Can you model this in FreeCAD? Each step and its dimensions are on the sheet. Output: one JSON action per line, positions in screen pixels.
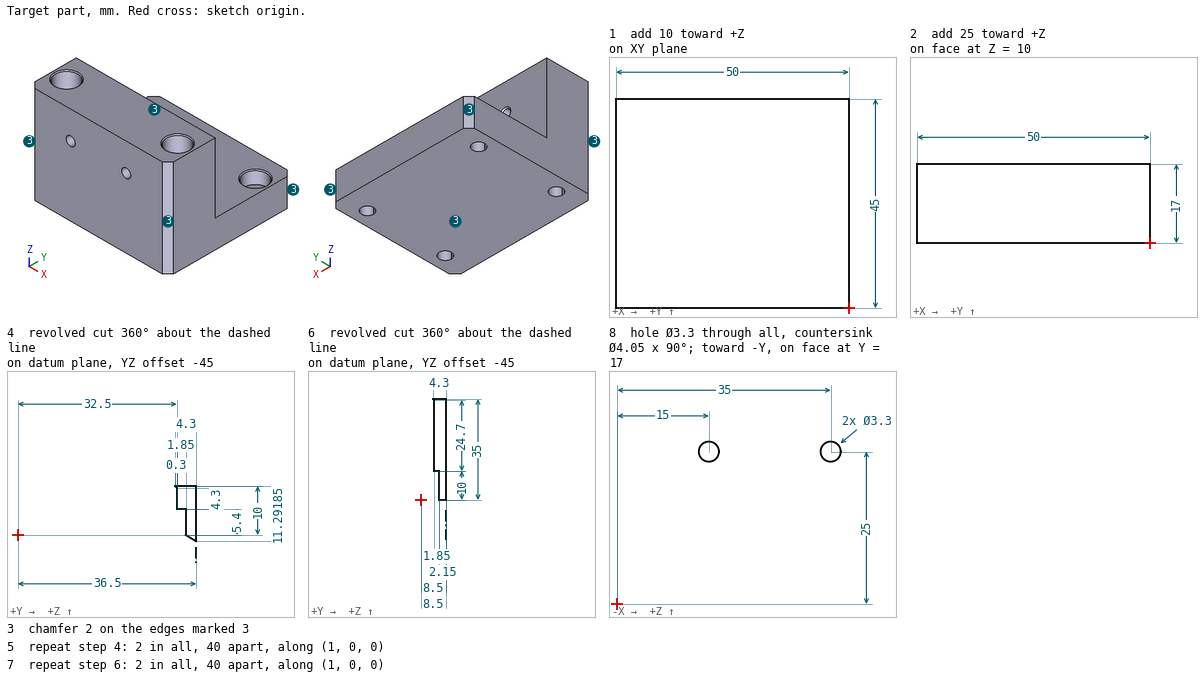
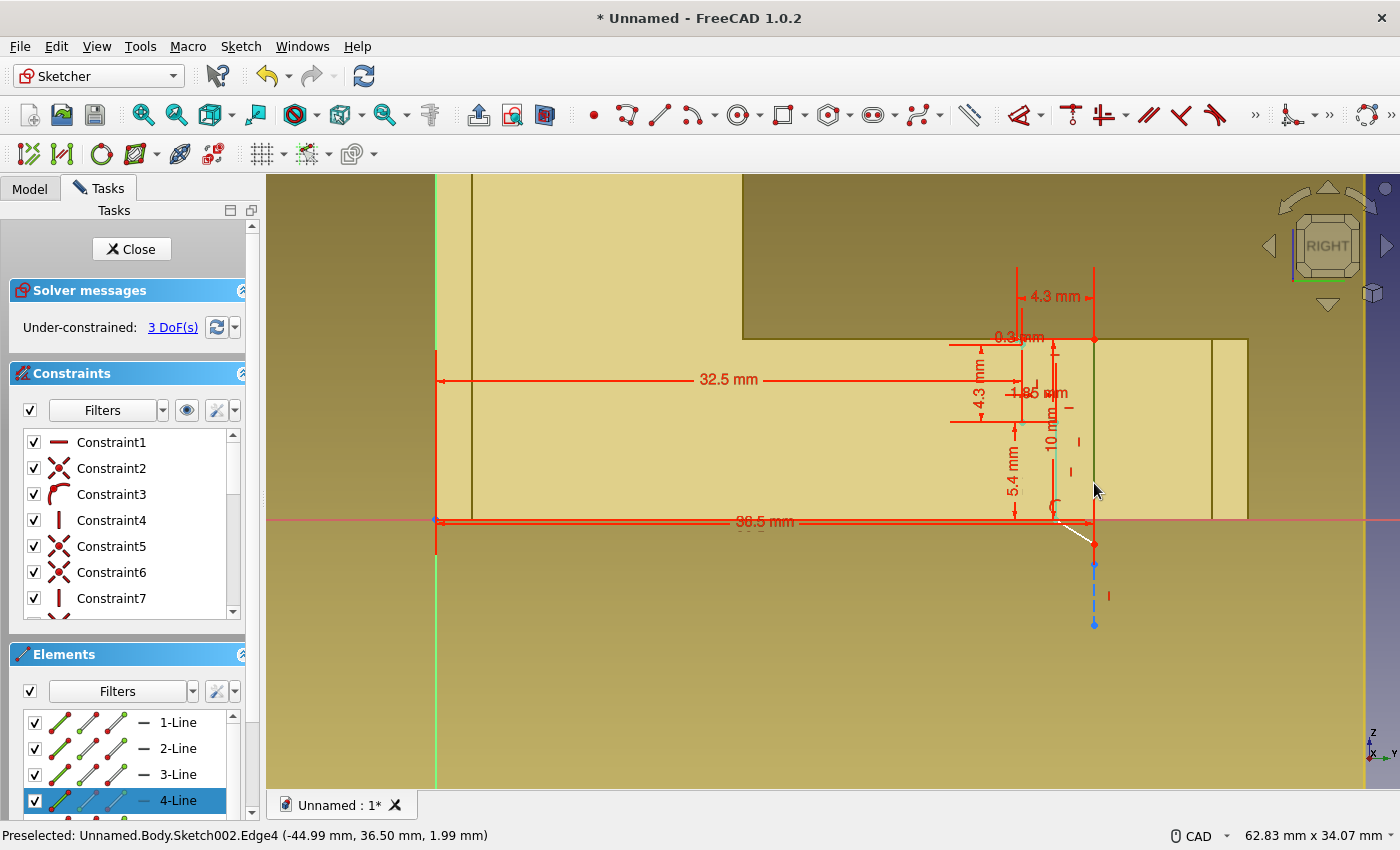
{"action": "left_click", "coordinate": [1040, 116]}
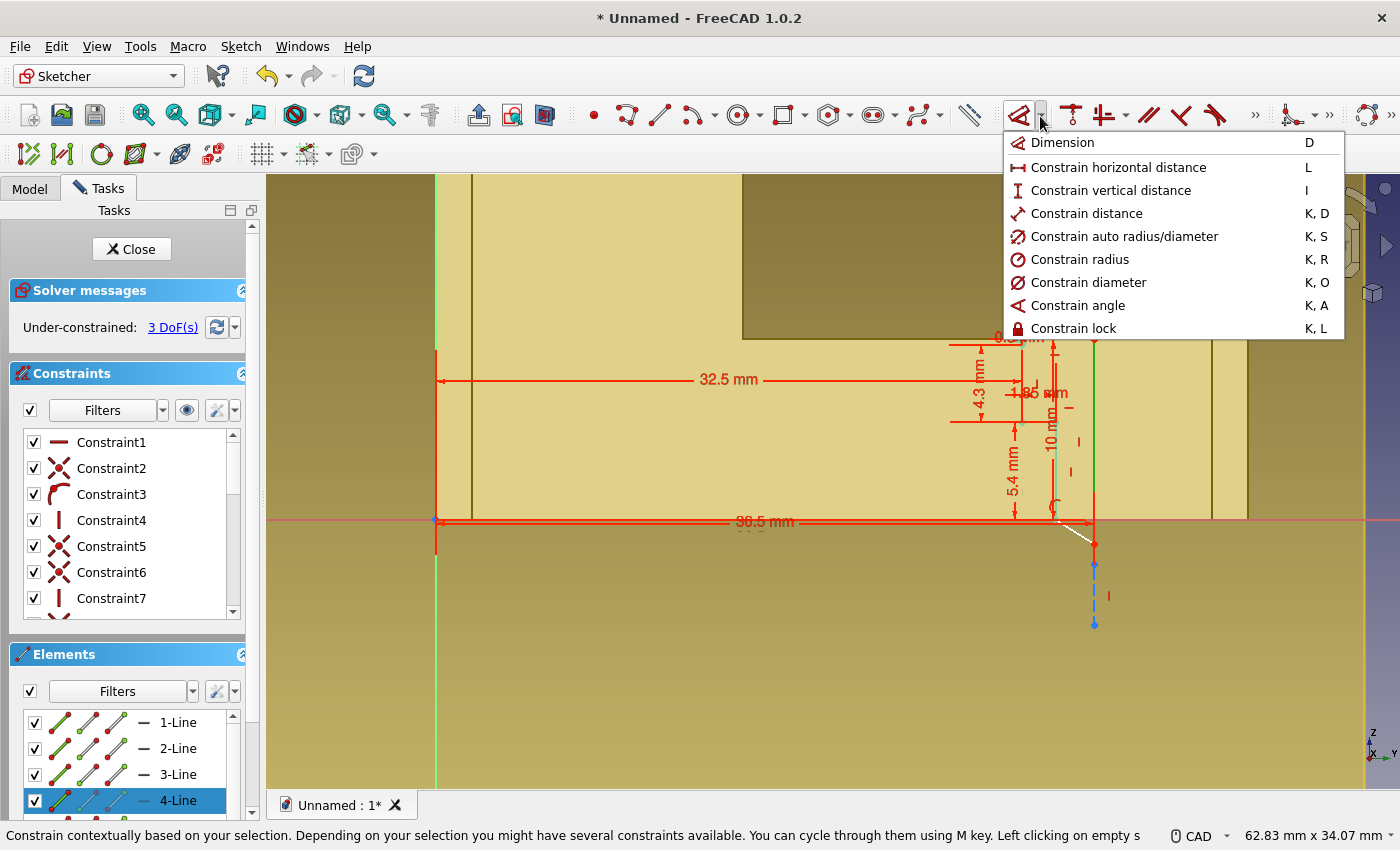
{"action": "left_click", "coordinate": [1174, 190]}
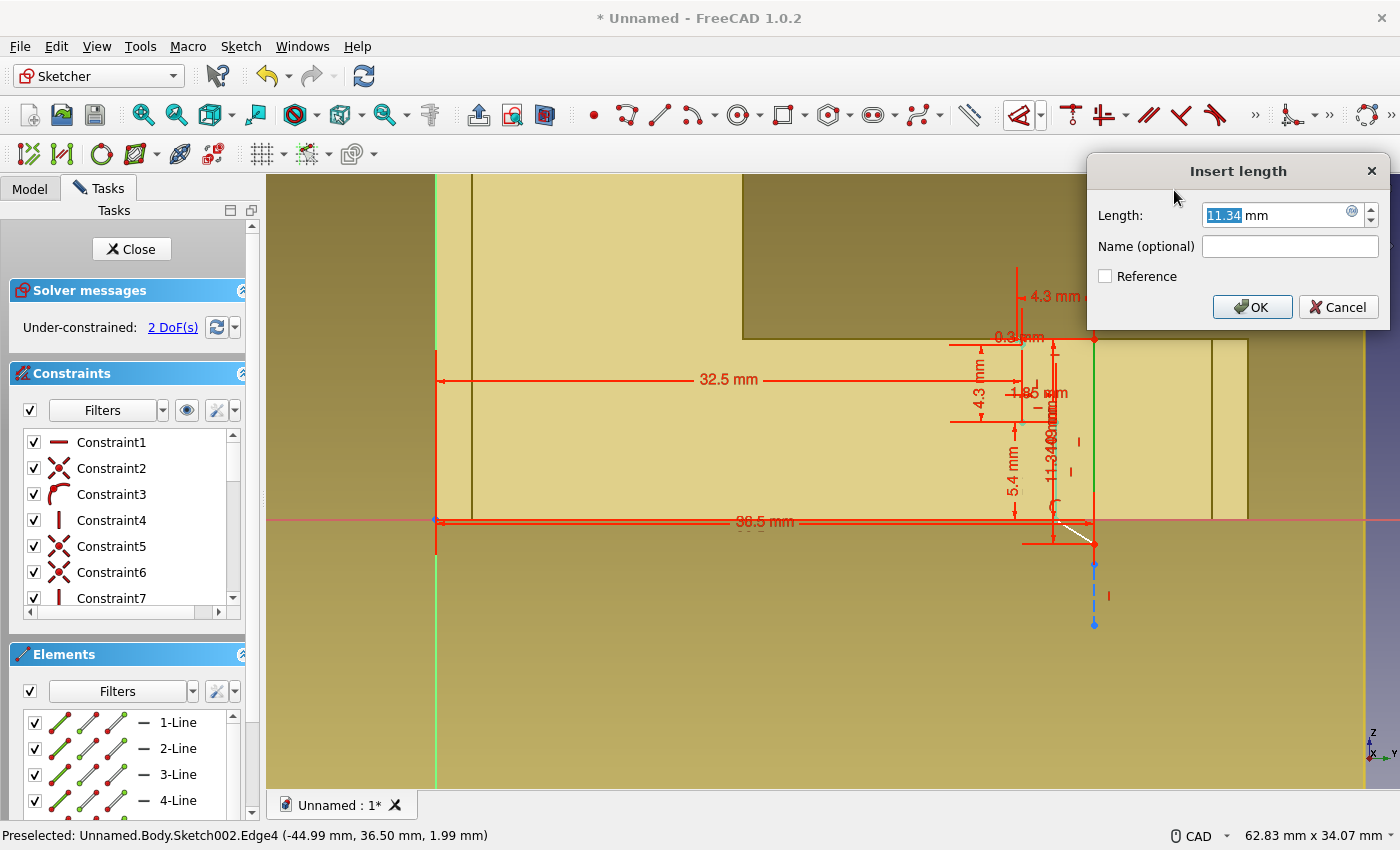
{"action": "type", "text": "11.29185"}
{"action": "key", "text": "Return"}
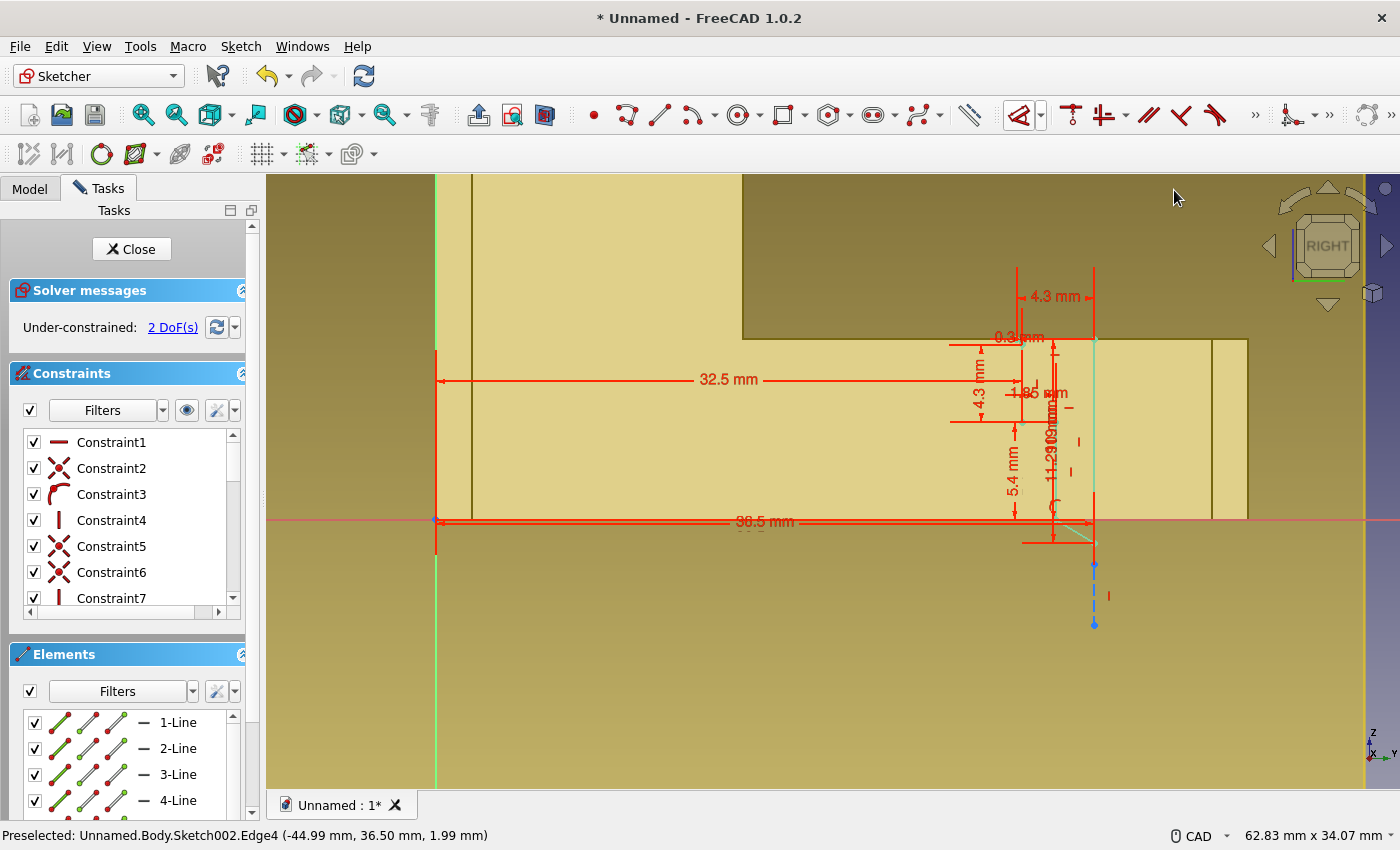
{"action": "left_click", "coordinate": [132, 249]}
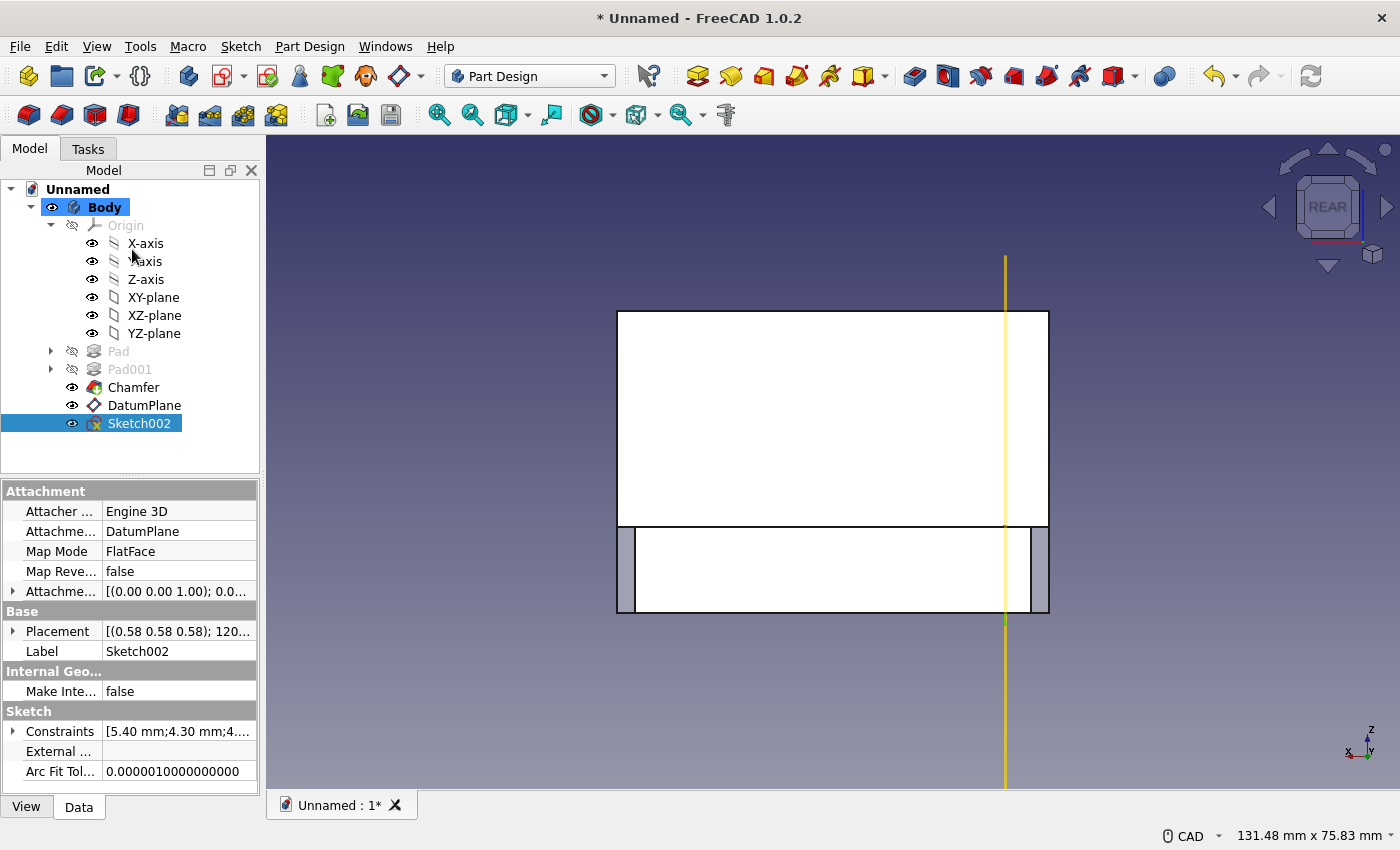
{"action": "left_click", "coordinate": [981, 76]}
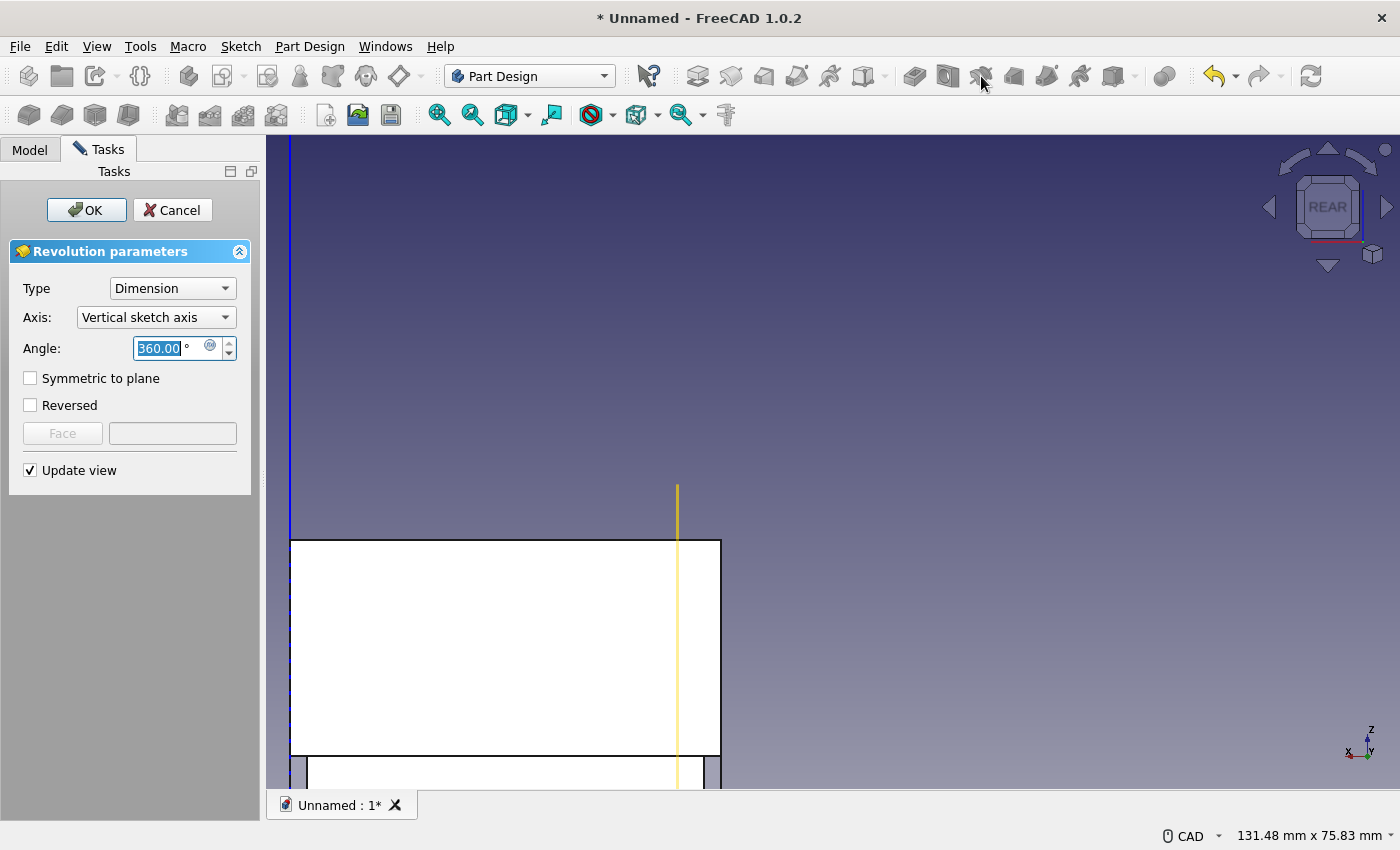
{"action": "left_click", "coordinate": [157, 318]}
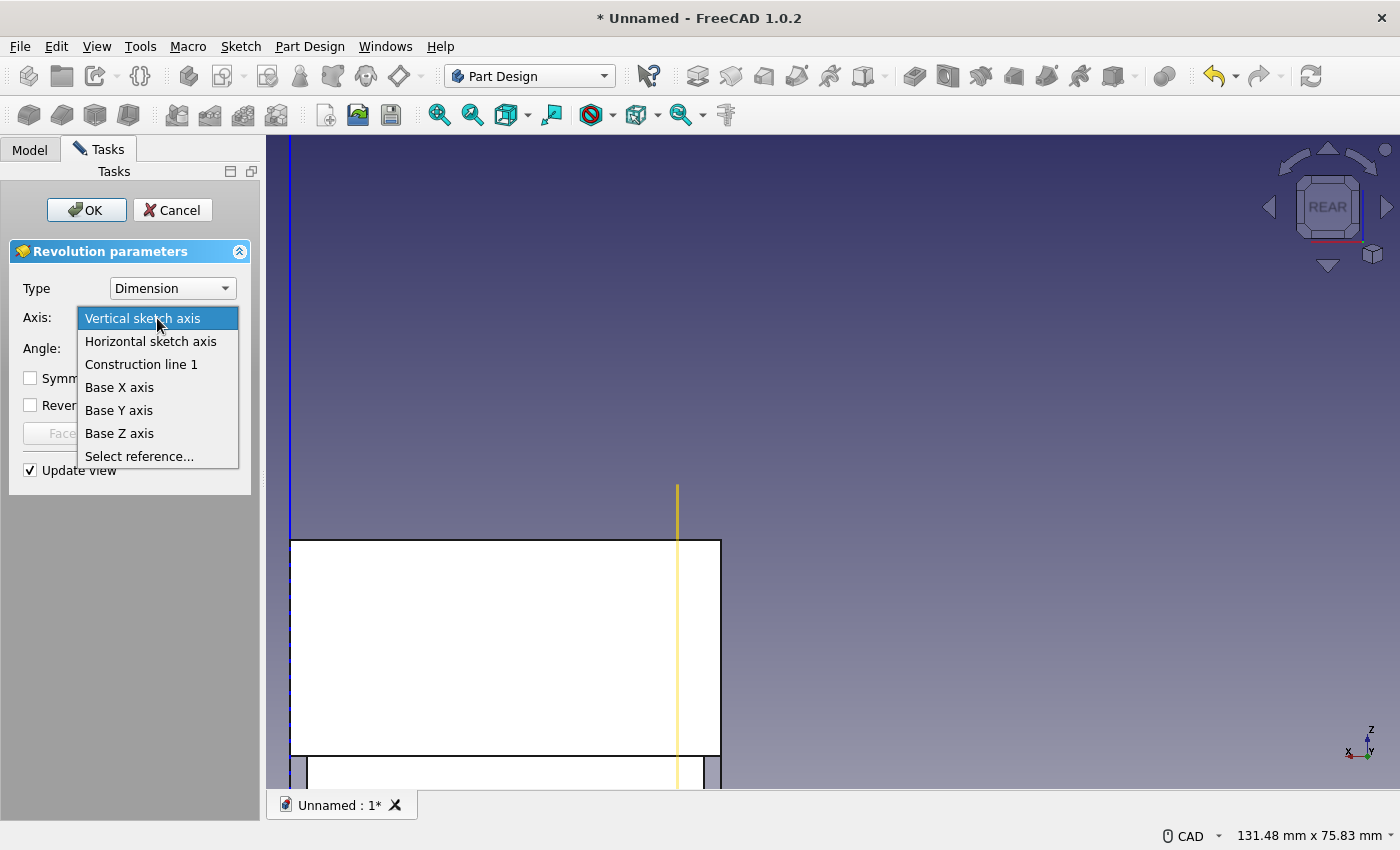
{"action": "left_click", "coordinate": [156, 364]}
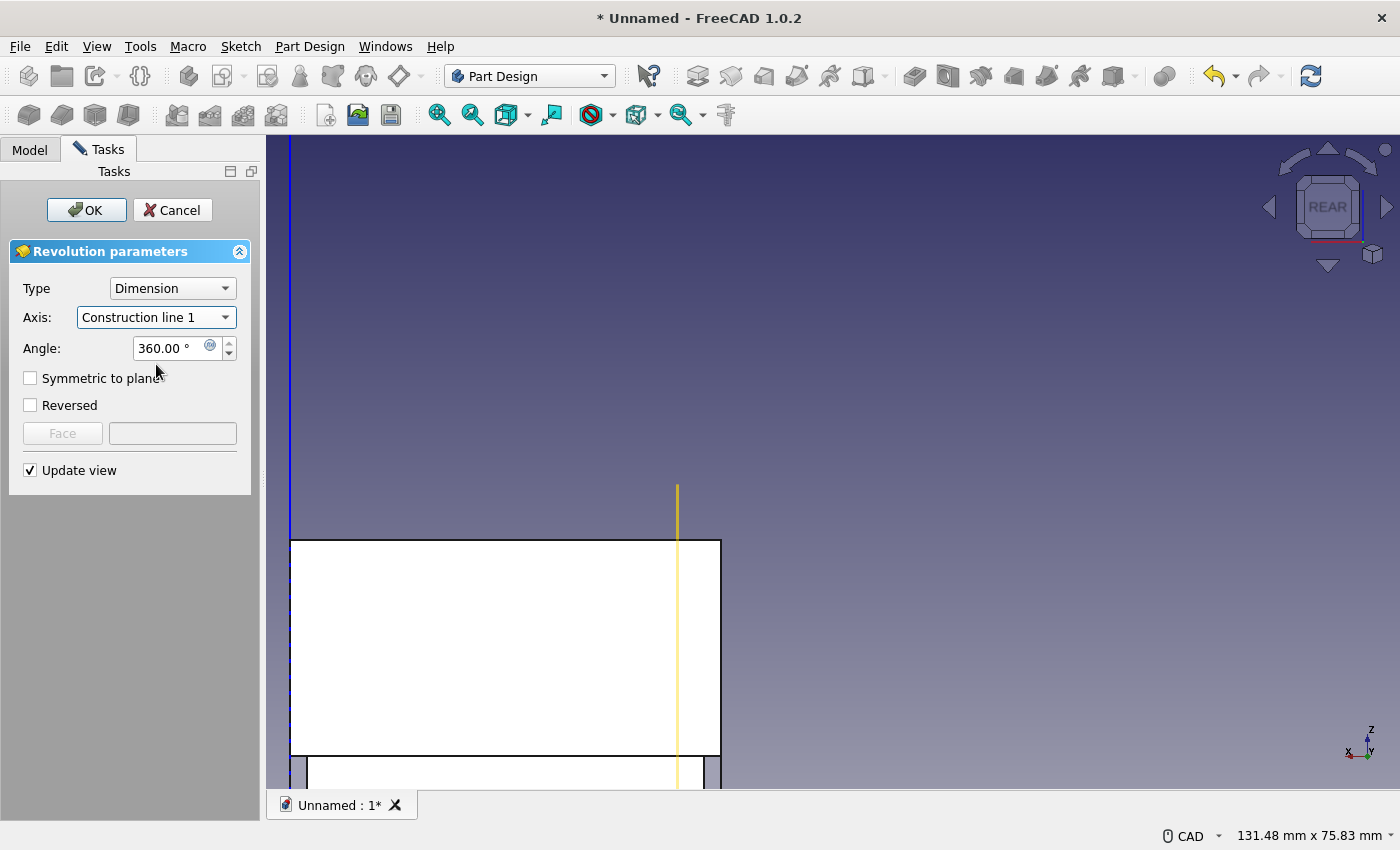
{"action": "left_click", "coordinate": [87, 210]}